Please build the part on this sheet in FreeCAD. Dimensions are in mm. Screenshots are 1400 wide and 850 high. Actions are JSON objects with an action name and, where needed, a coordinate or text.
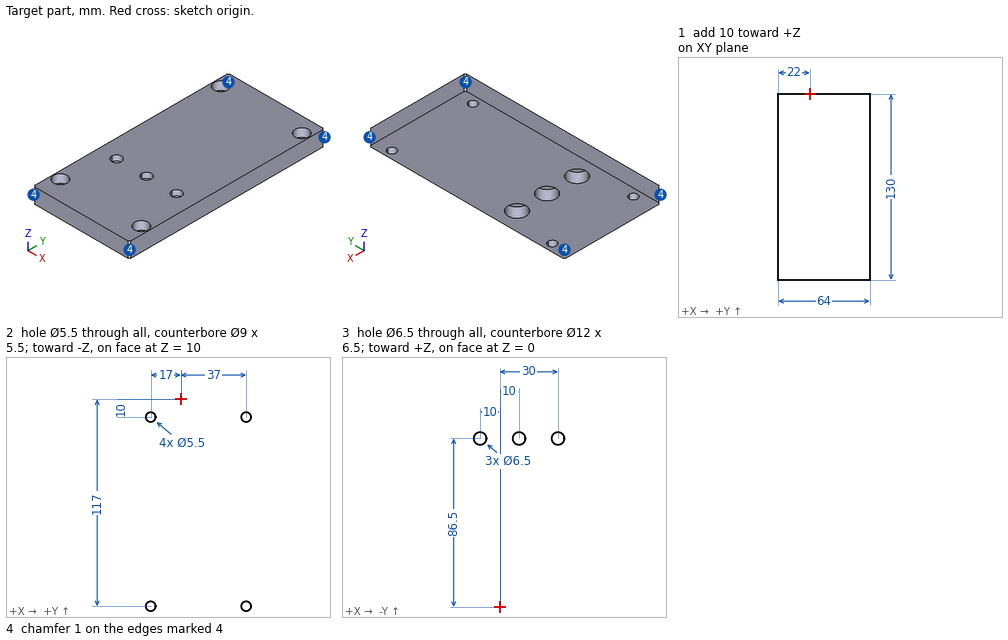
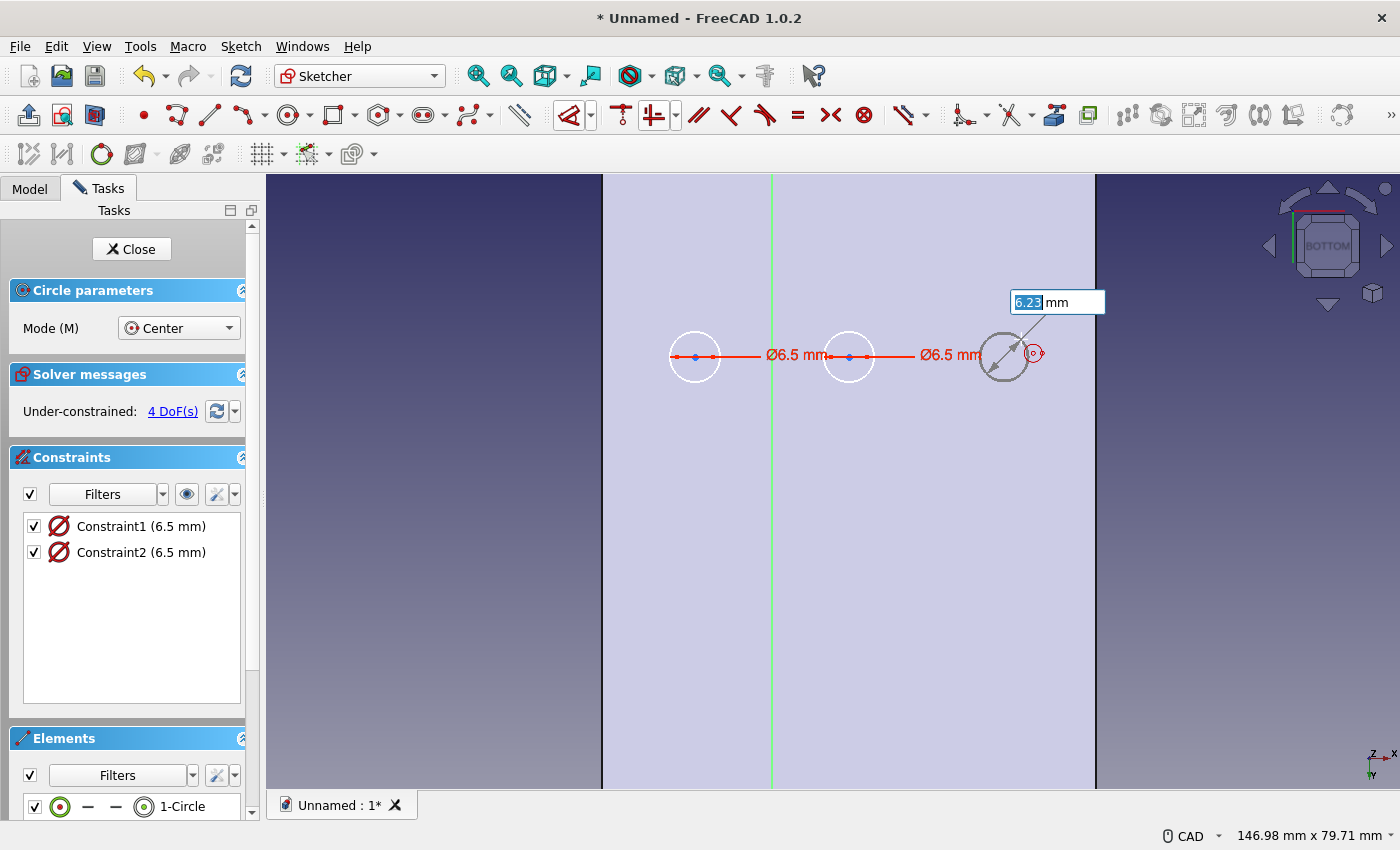
{"action": "type", "text": "6.5"}
{"action": "key", "text": "Return"}
{"action": "key", "text": "Escape"}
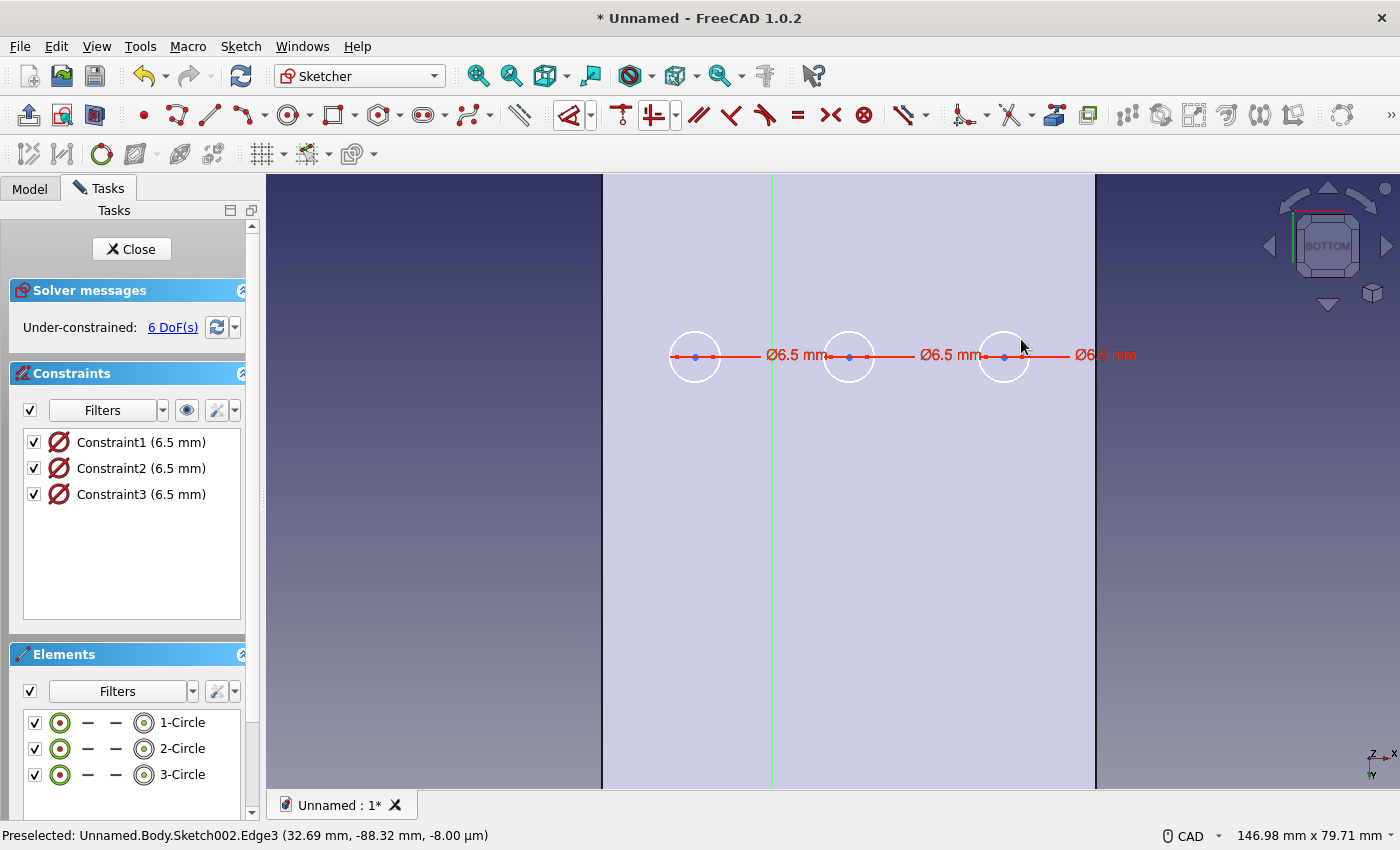
{"action": "left_click", "coordinate": [695, 357]}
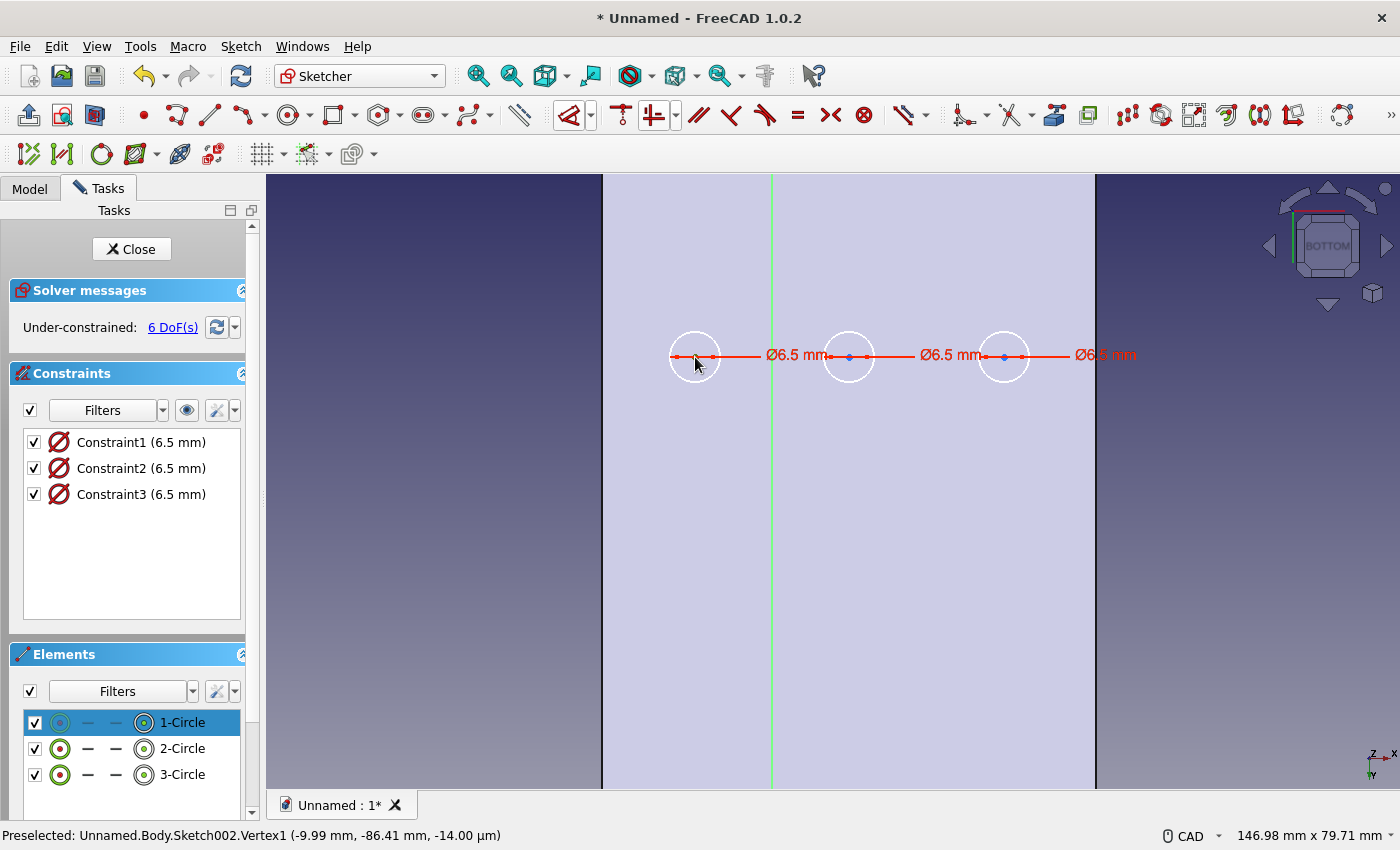
{"action": "left_click", "coordinate": [849, 357]}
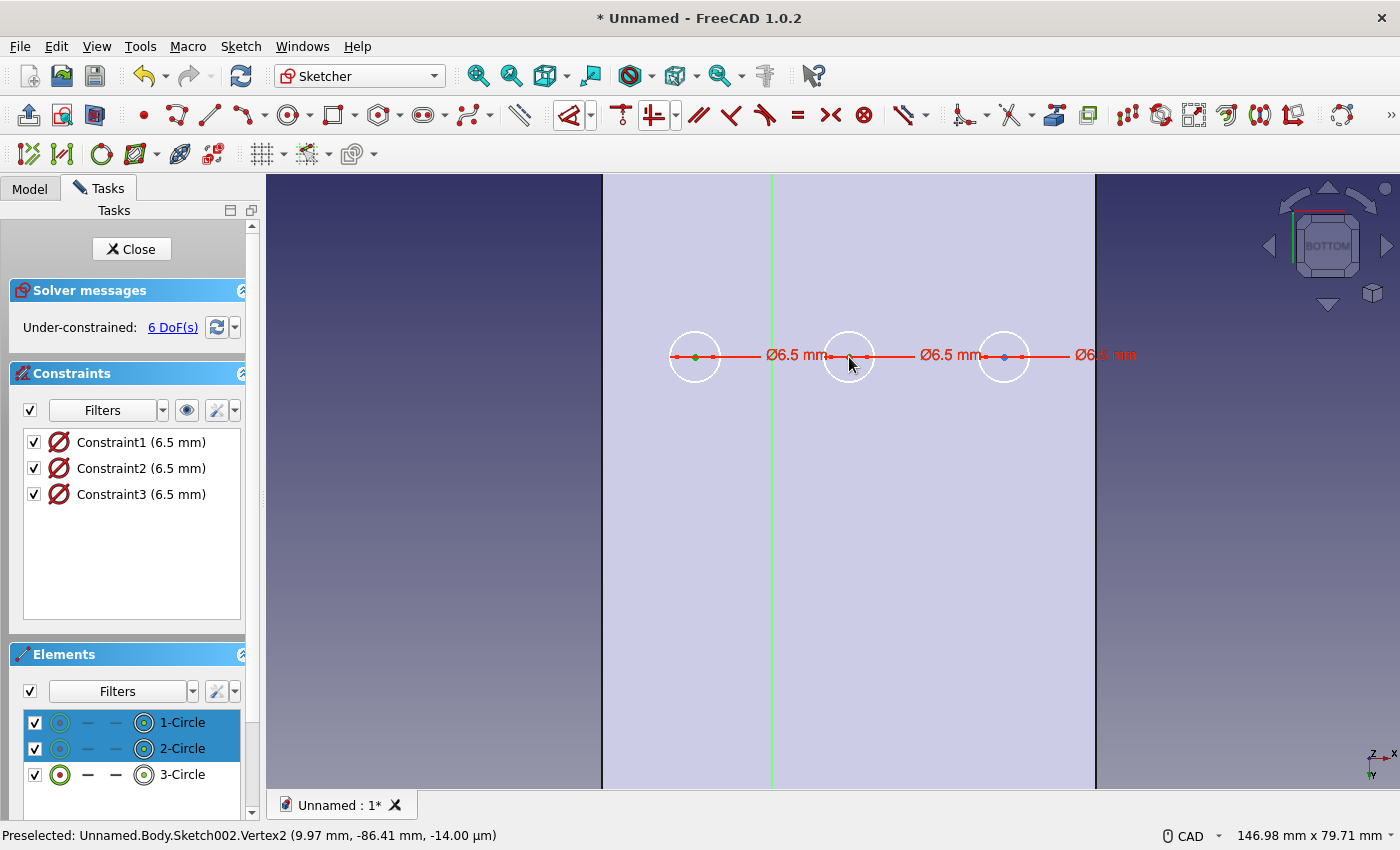
{"action": "key", "text": "h"}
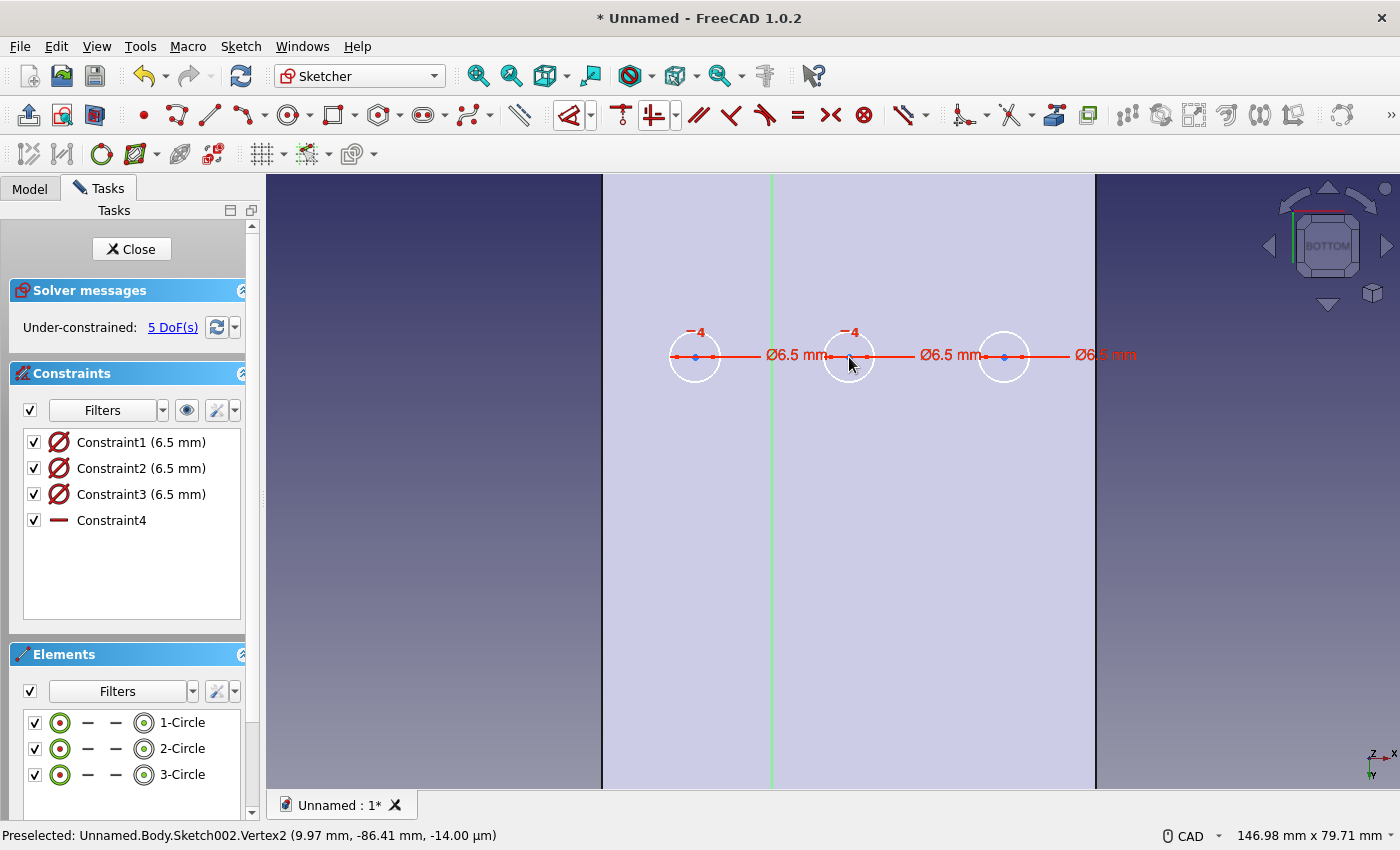
{"action": "left_click", "coordinate": [849, 357]}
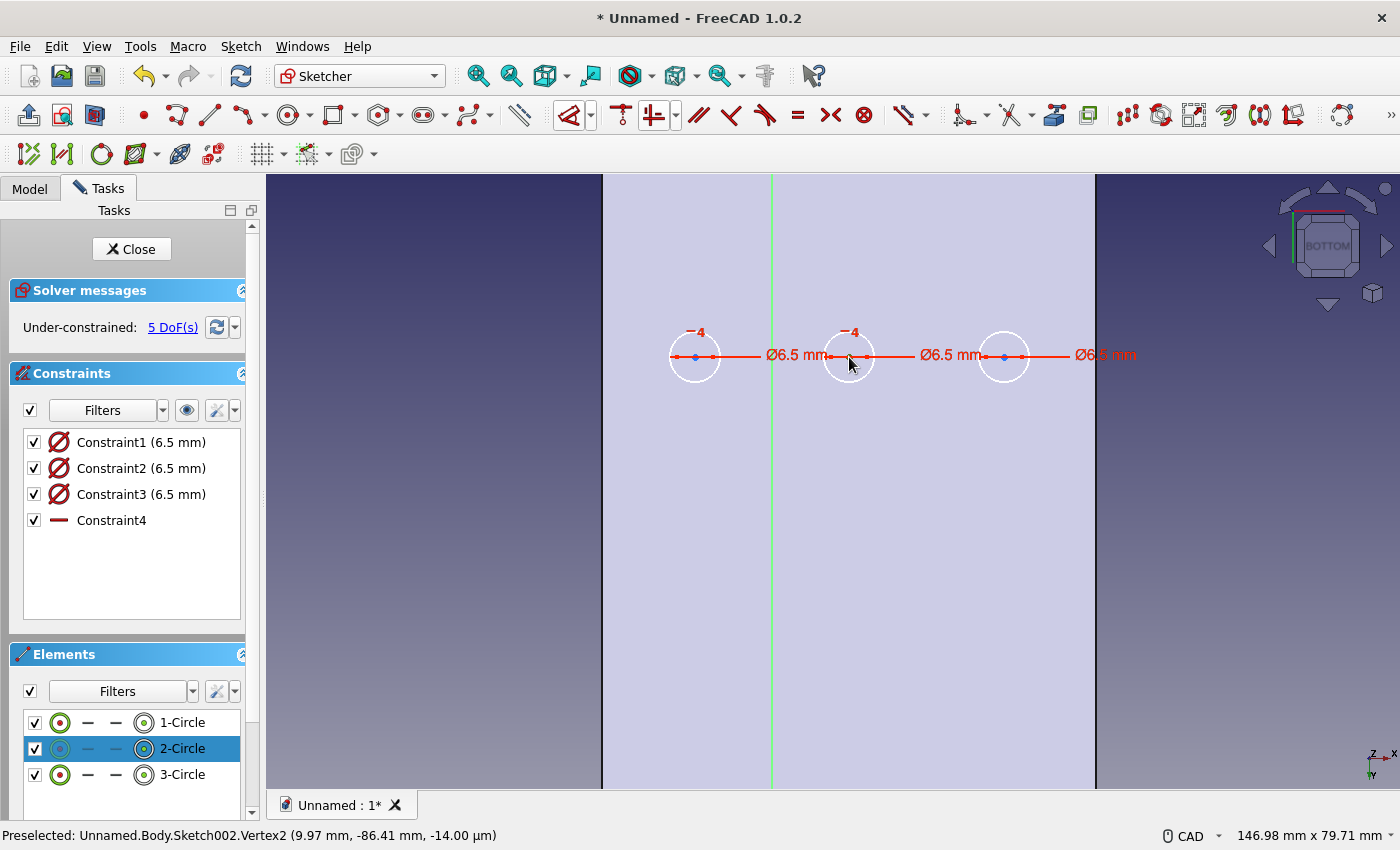
{"action": "left_click", "coordinate": [1004, 357]}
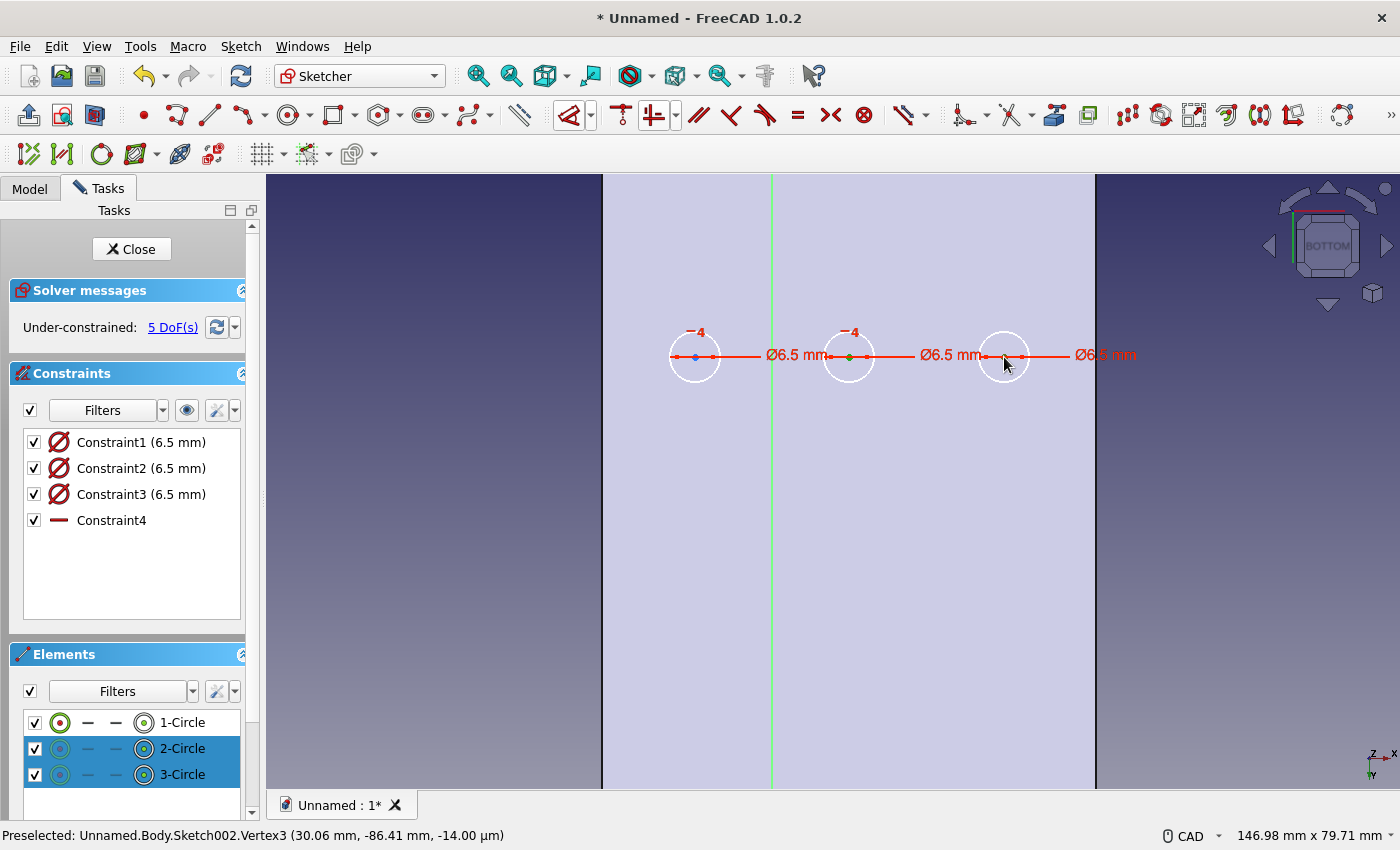
{"action": "key", "text": "h"}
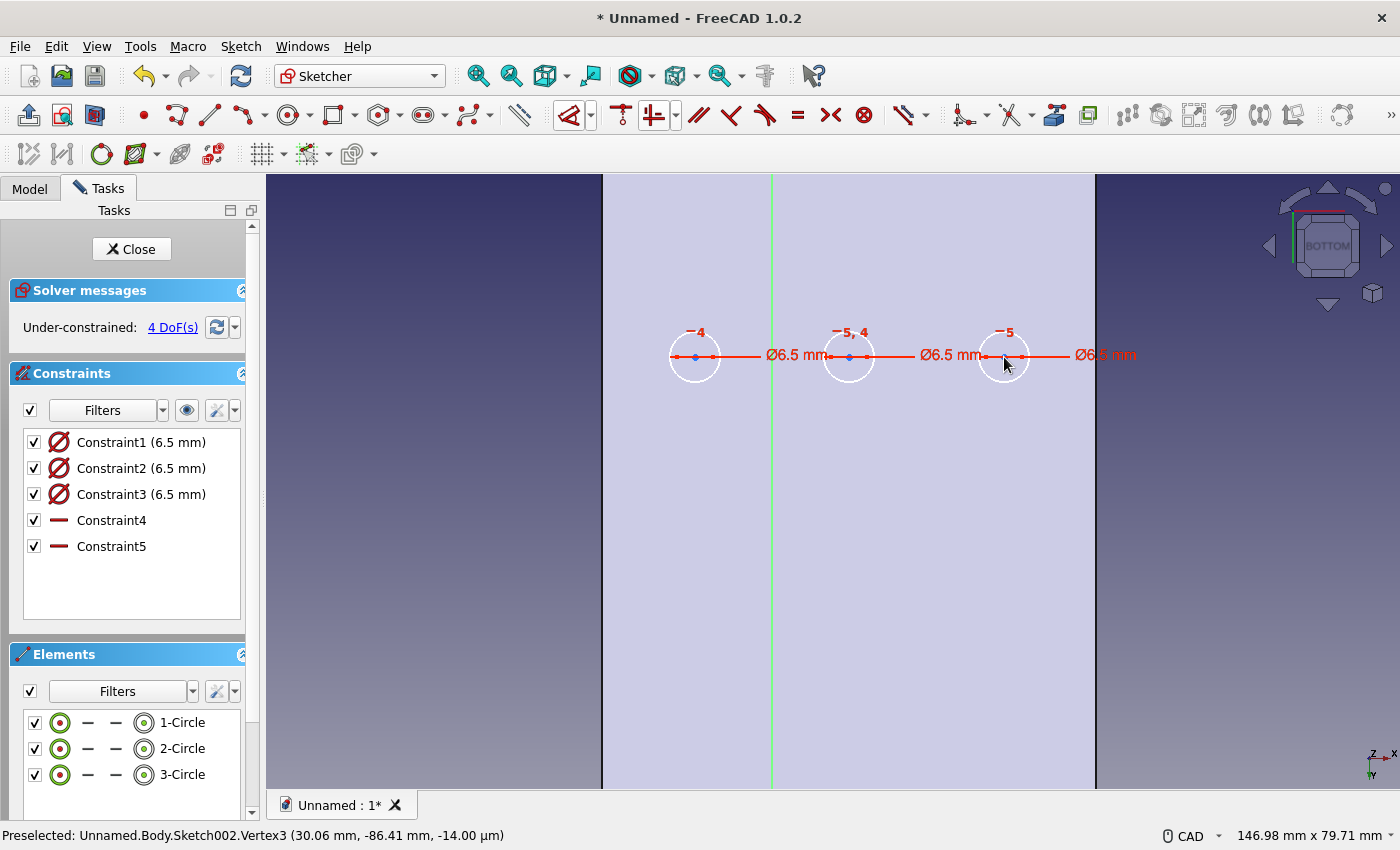
{"action": "left_click", "coordinate": [695, 357]}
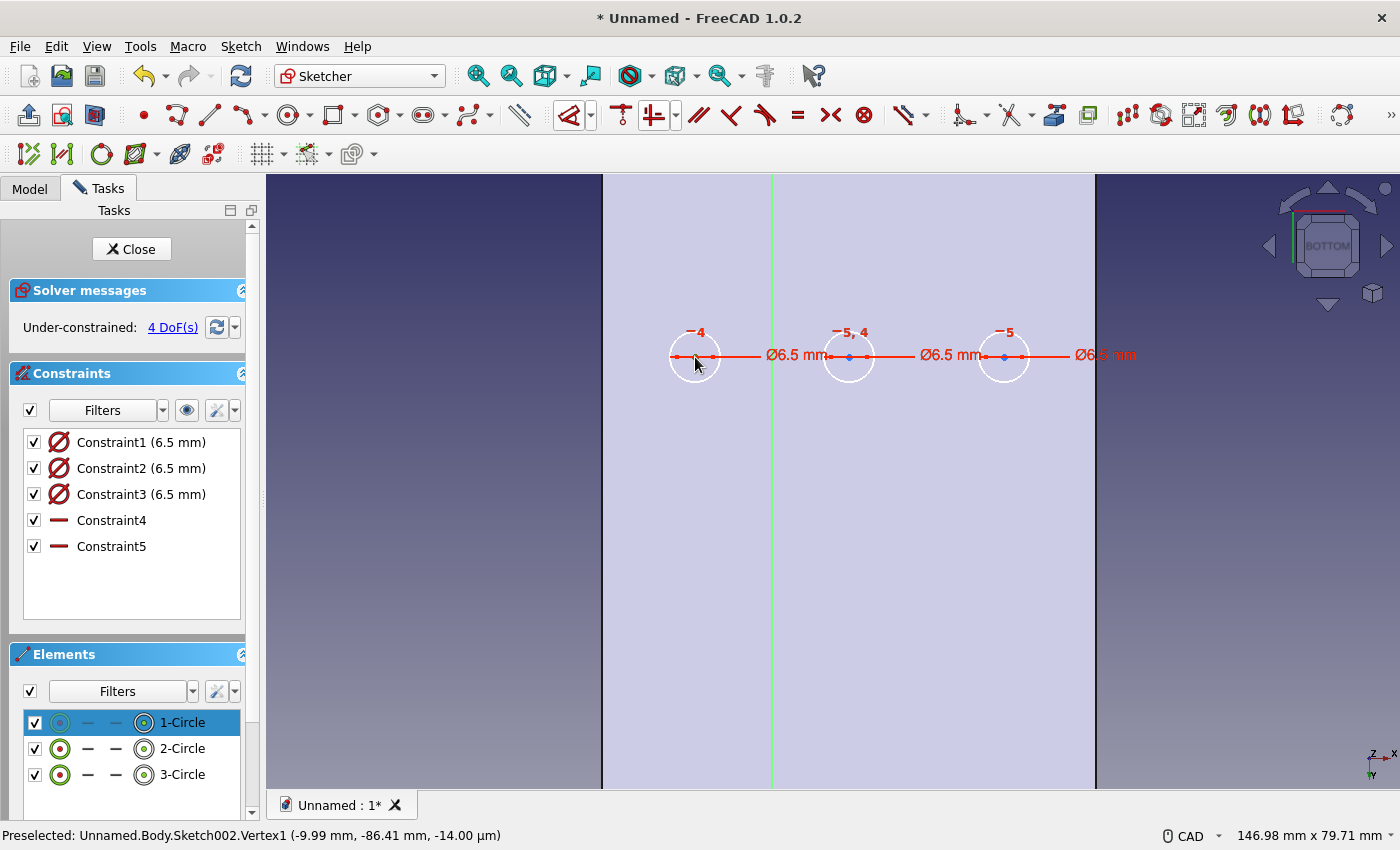
{"action": "key", "text": "l"}